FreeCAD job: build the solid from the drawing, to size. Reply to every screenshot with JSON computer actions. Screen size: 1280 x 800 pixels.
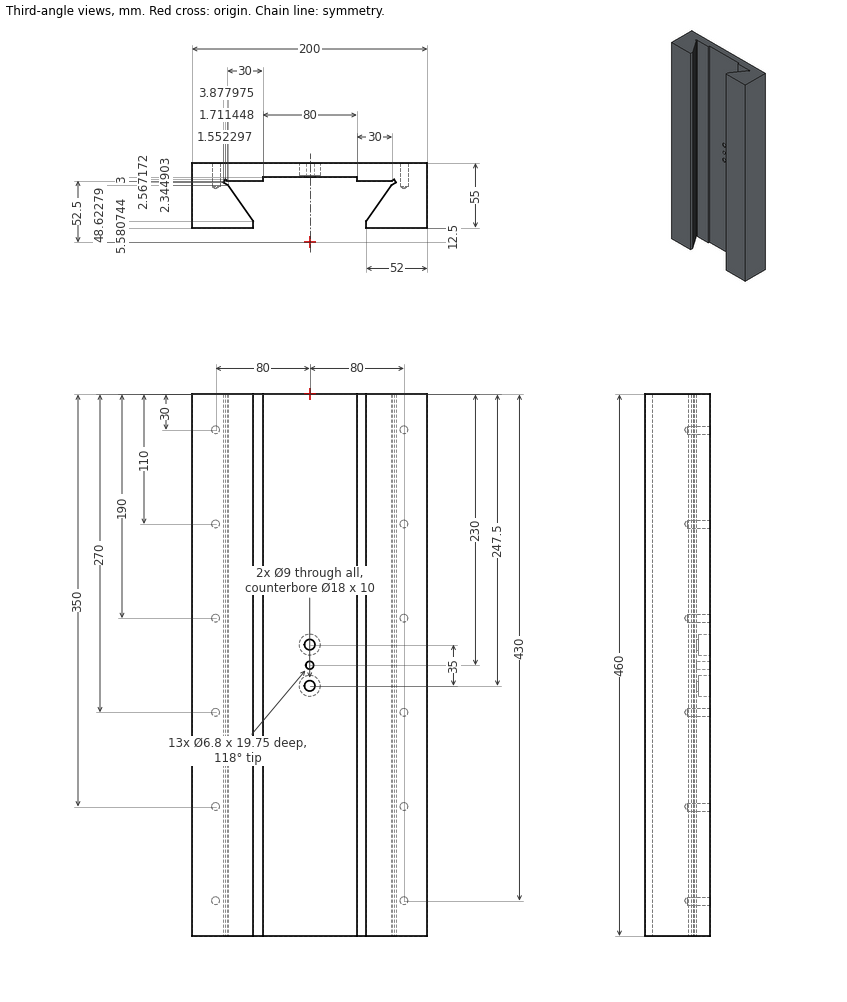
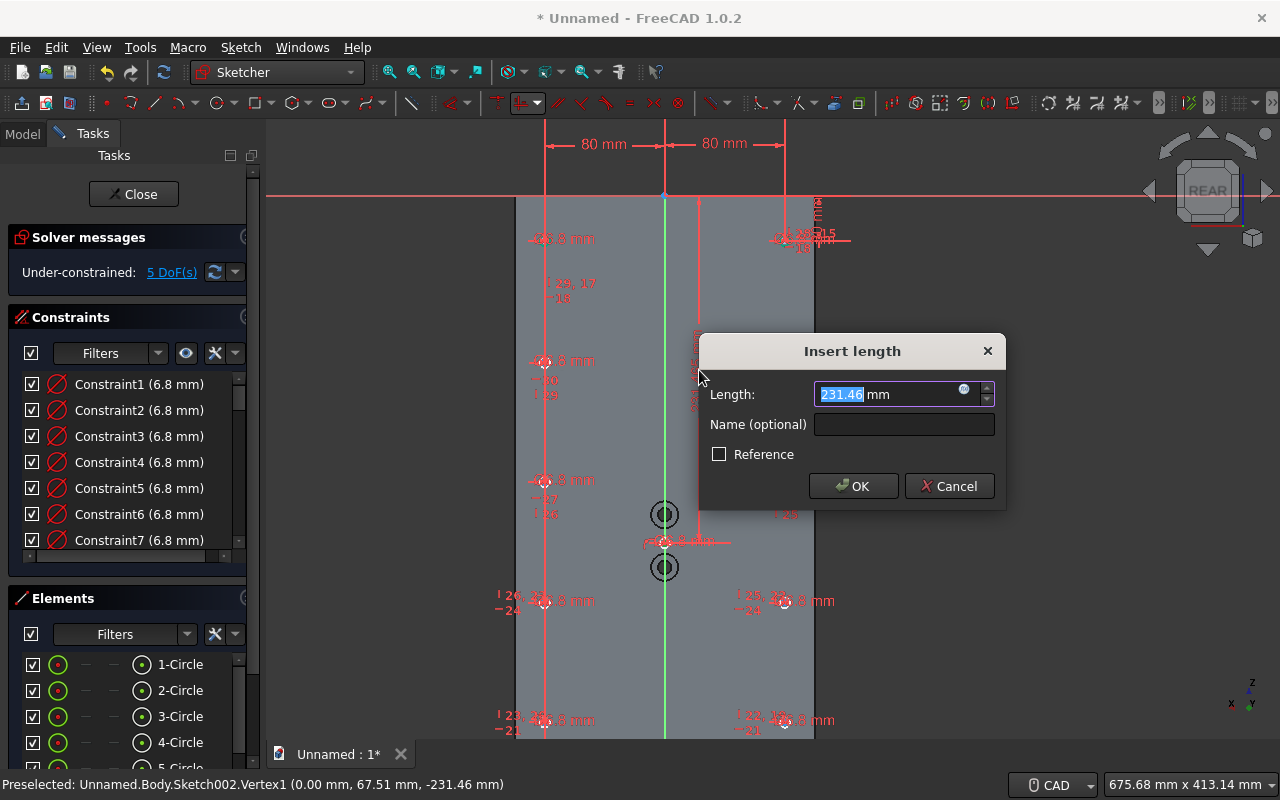
{"action": "type", "text": "230"}
{"action": "key", "text": "Return"}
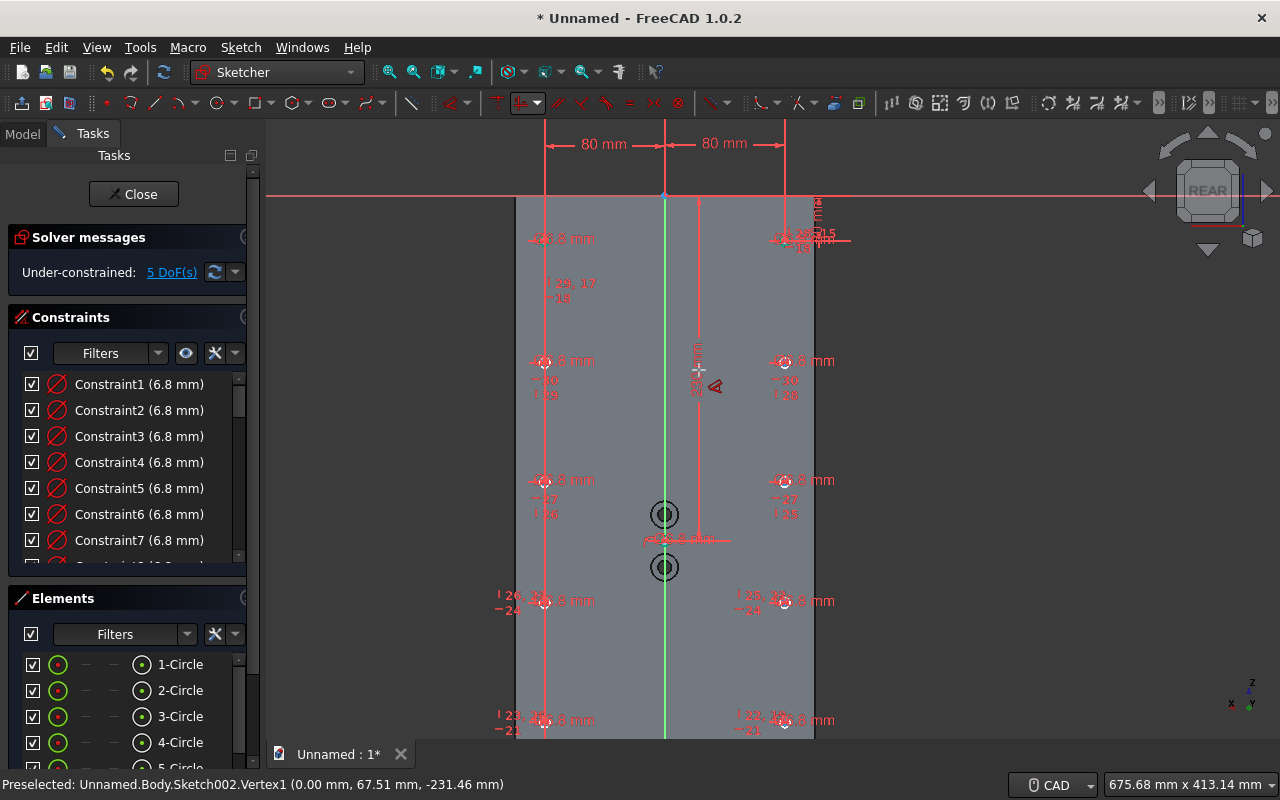
{"action": "scroll", "coordinate": [786, 242], "scroll_direction": "down", "scroll_amount": 2}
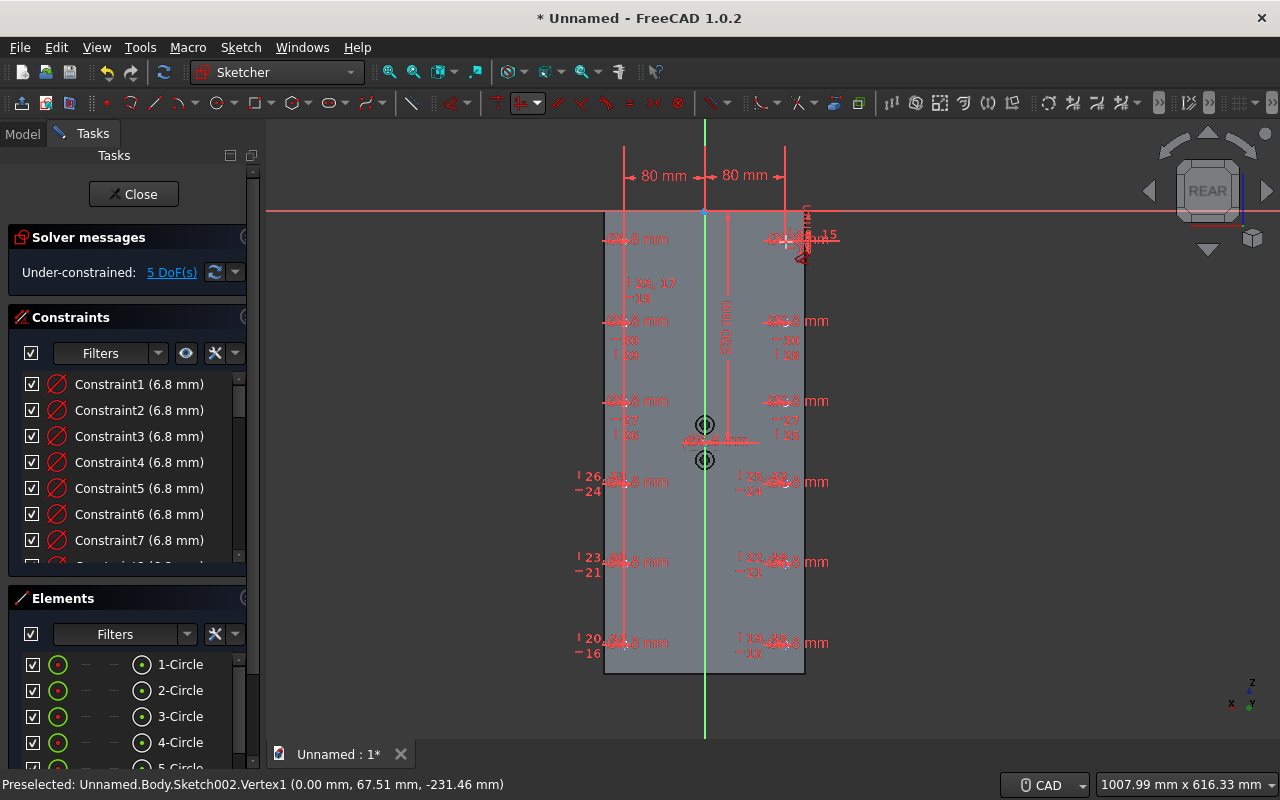
{"action": "left_click", "coordinate": [624, 645]}
{"action": "left_click", "coordinate": [590, 428]}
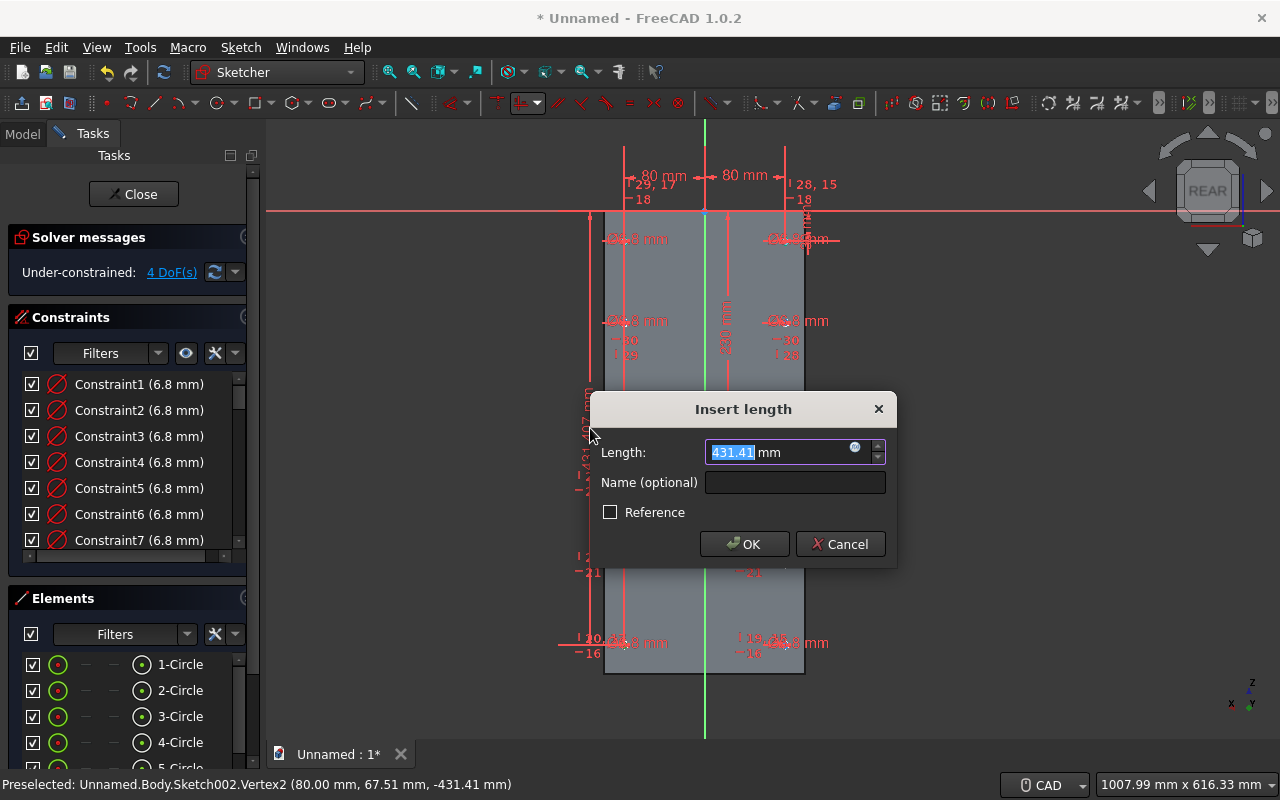
{"action": "type", "text": "430"}
{"action": "key", "text": "Return"}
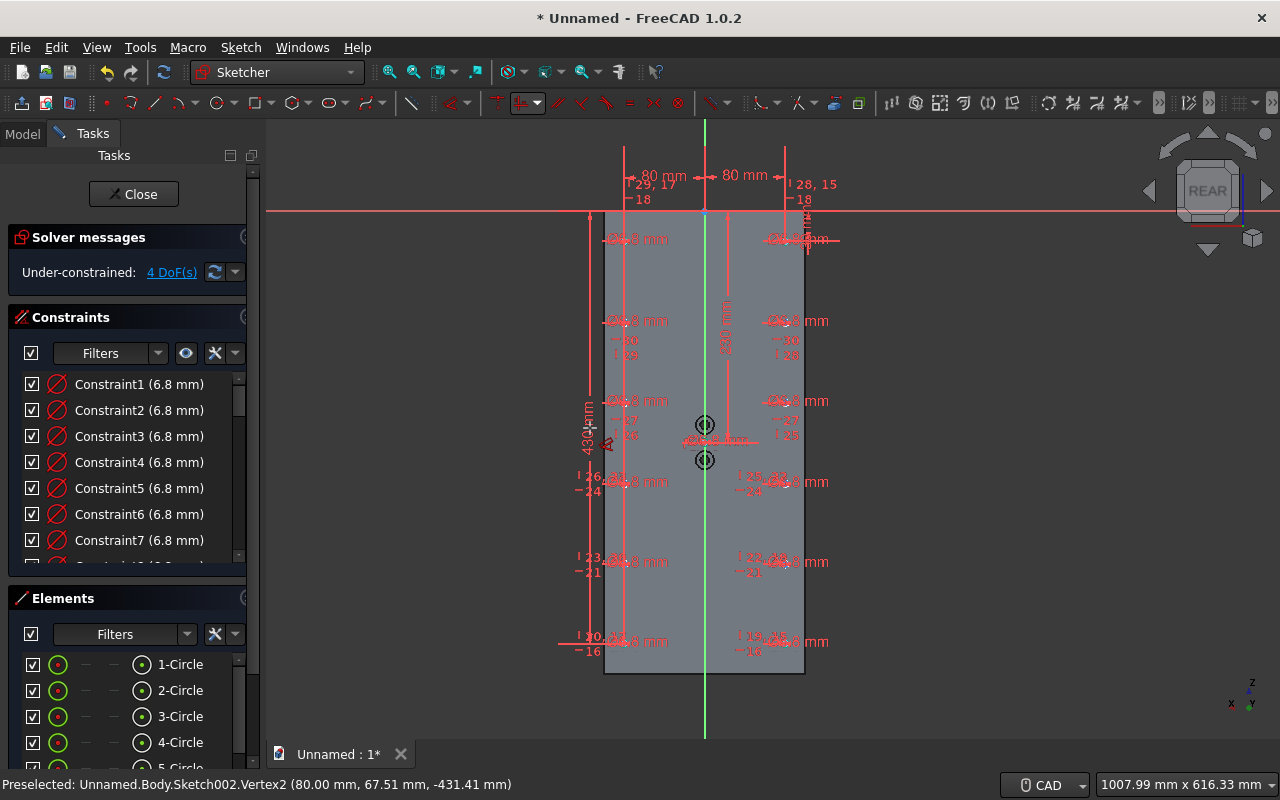
{"action": "left_click", "coordinate": [785, 564]}
{"action": "left_click", "coordinate": [819, 388]}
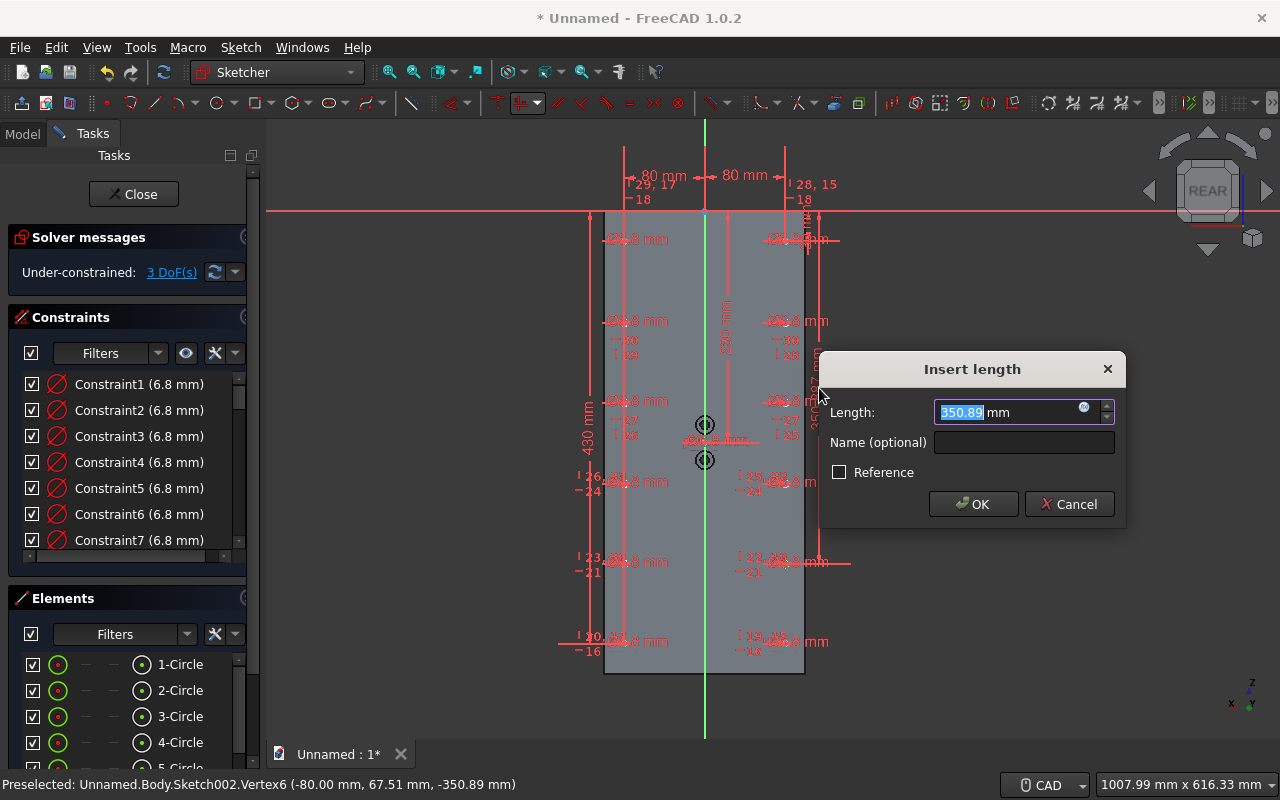
{"action": "type", "text": "350"}
{"action": "key", "text": "Return"}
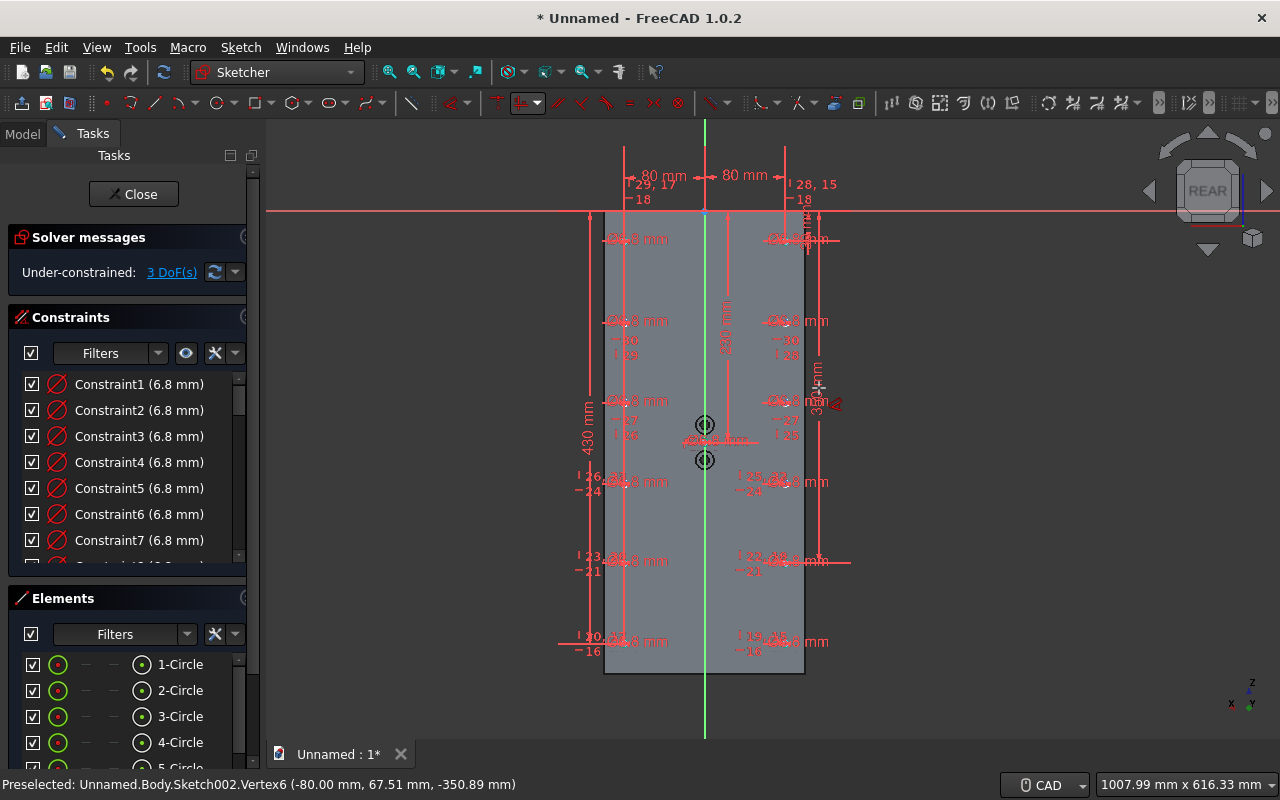
{"action": "left_click", "coordinate": [785, 484]}
{"action": "left_click", "coordinate": [819, 348]}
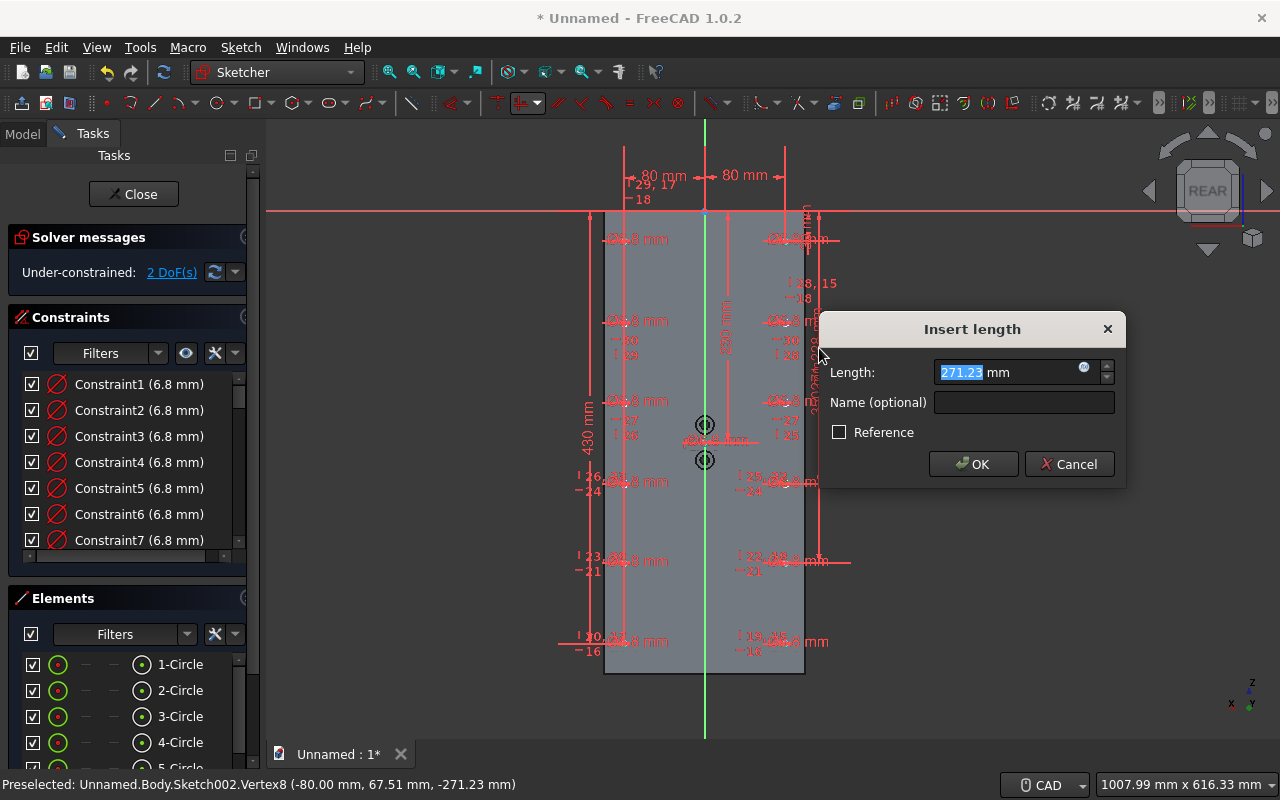
{"action": "type", "text": "270"}
{"action": "key", "text": "Return"}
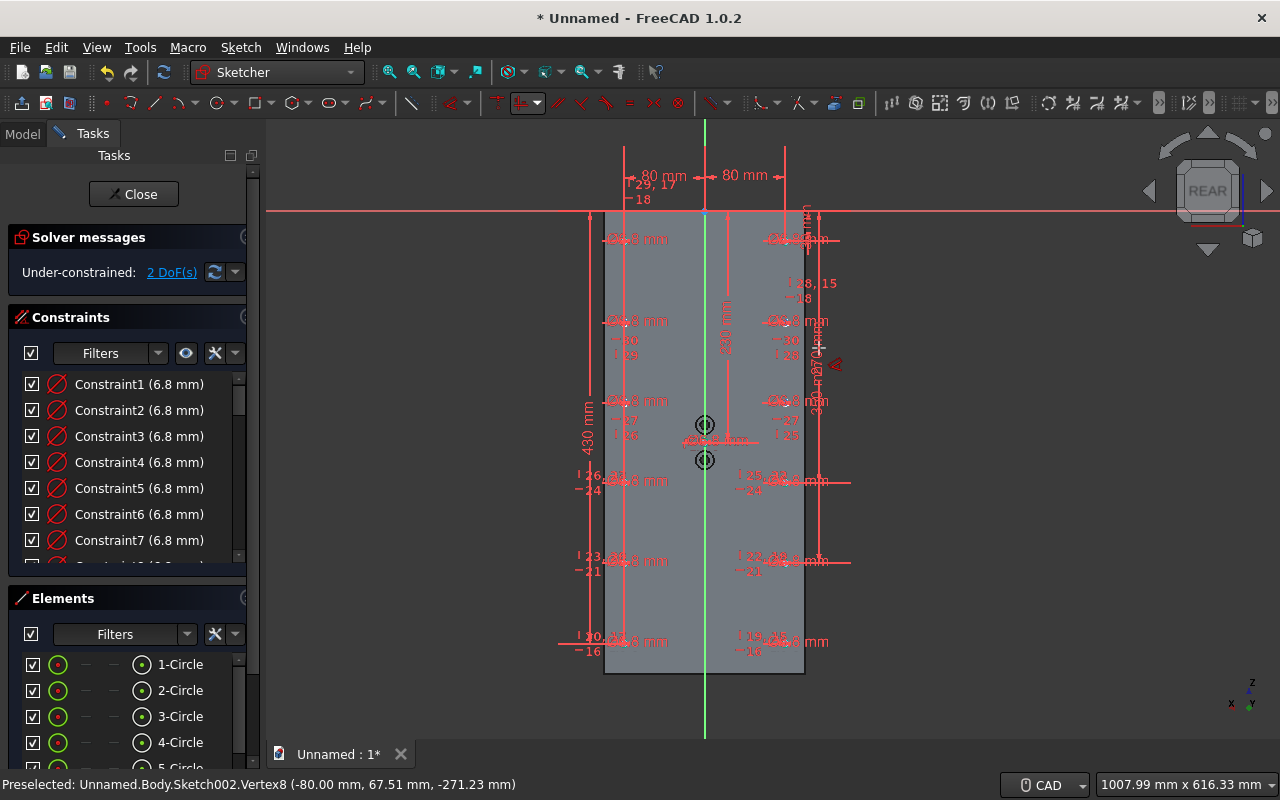
{"action": "left_click", "coordinate": [785, 403]}
{"action": "left_click", "coordinate": [819, 307]}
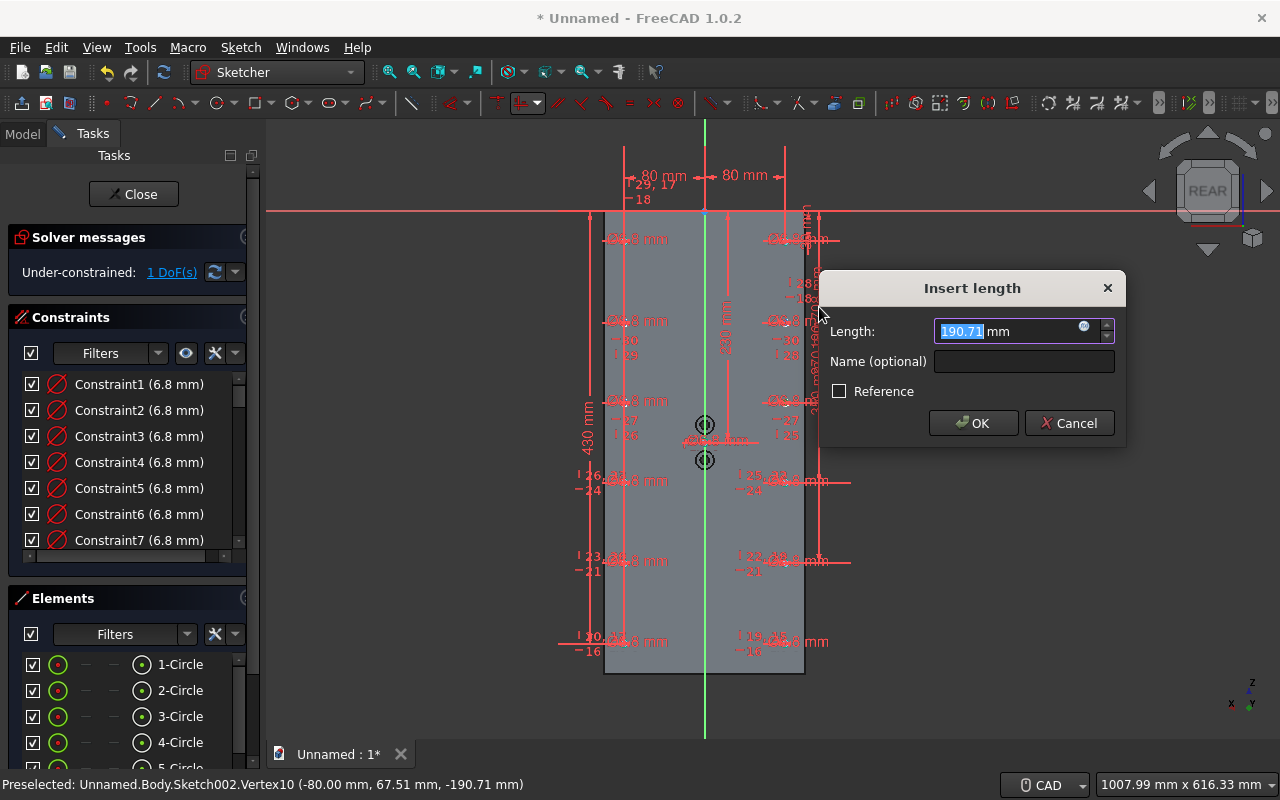
{"action": "type", "text": "190"}
{"action": "key", "text": "Return"}